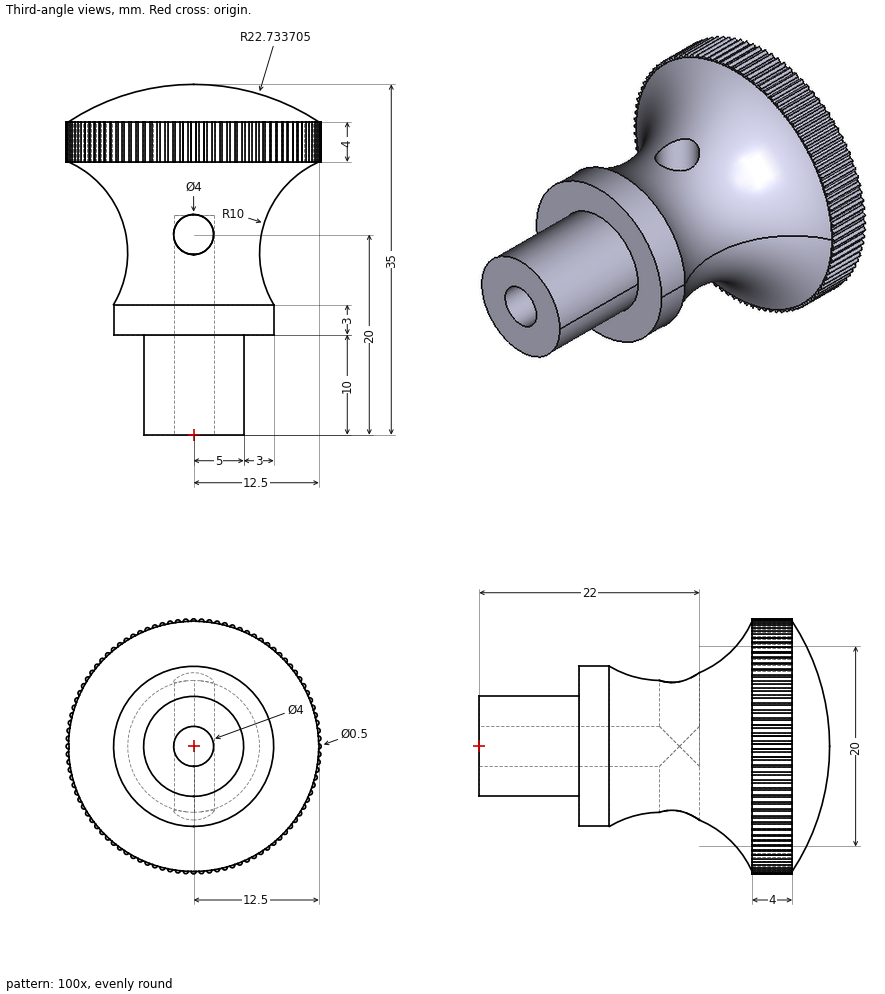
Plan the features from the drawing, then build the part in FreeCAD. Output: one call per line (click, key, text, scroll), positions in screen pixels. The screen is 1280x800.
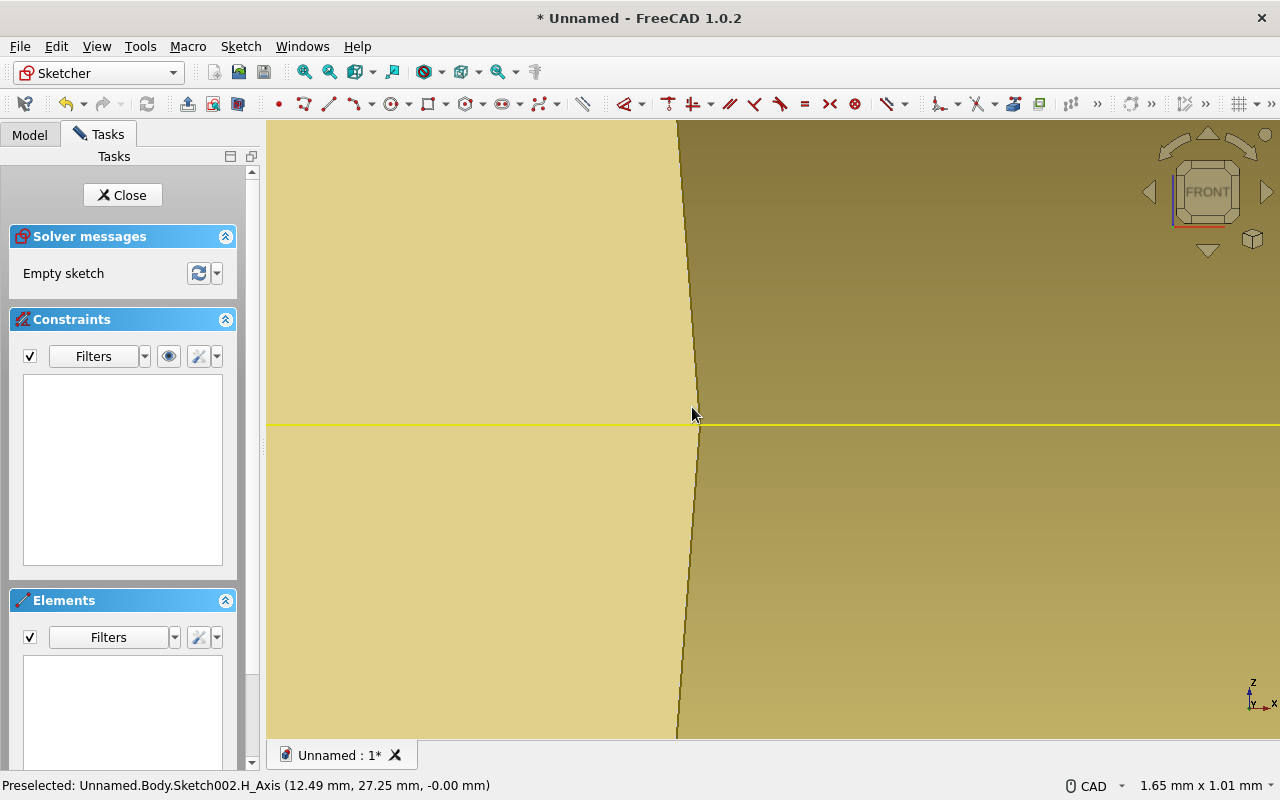
click(390, 104)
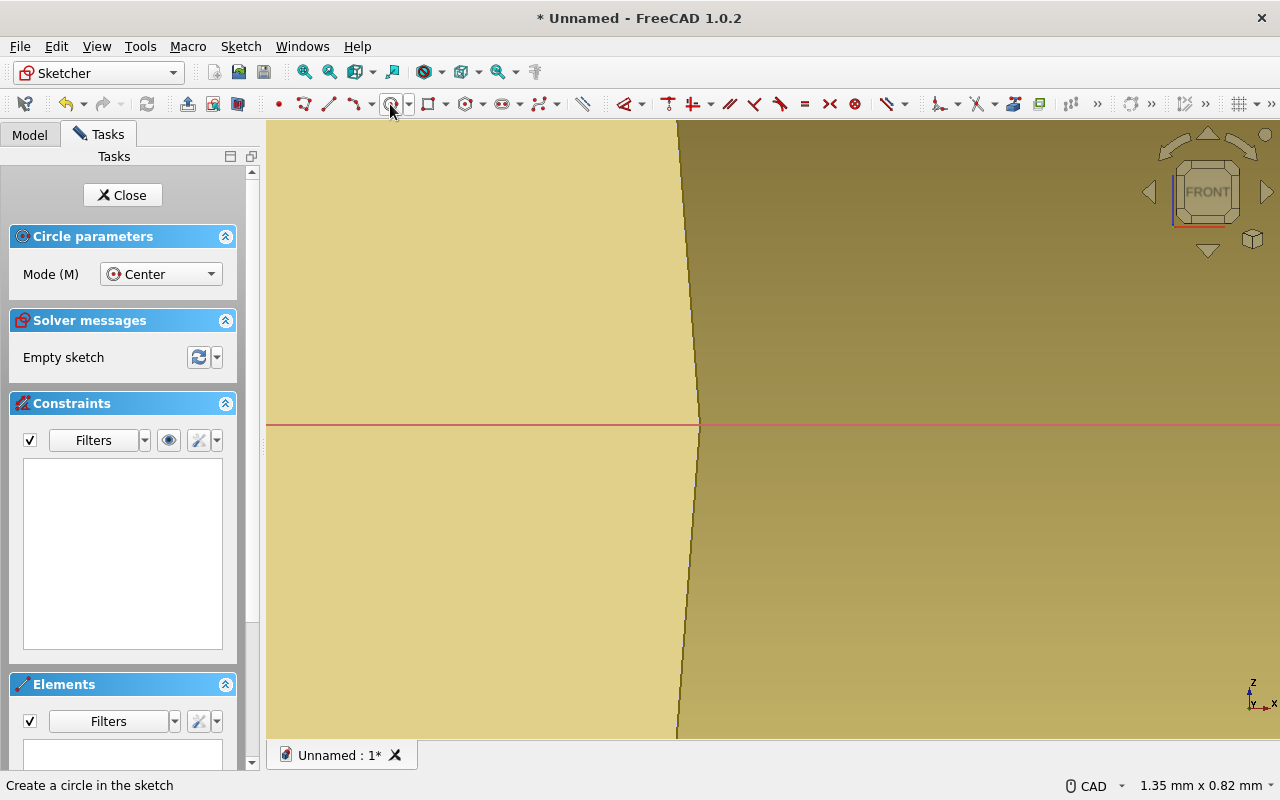
click(700, 425)
move(833, 292)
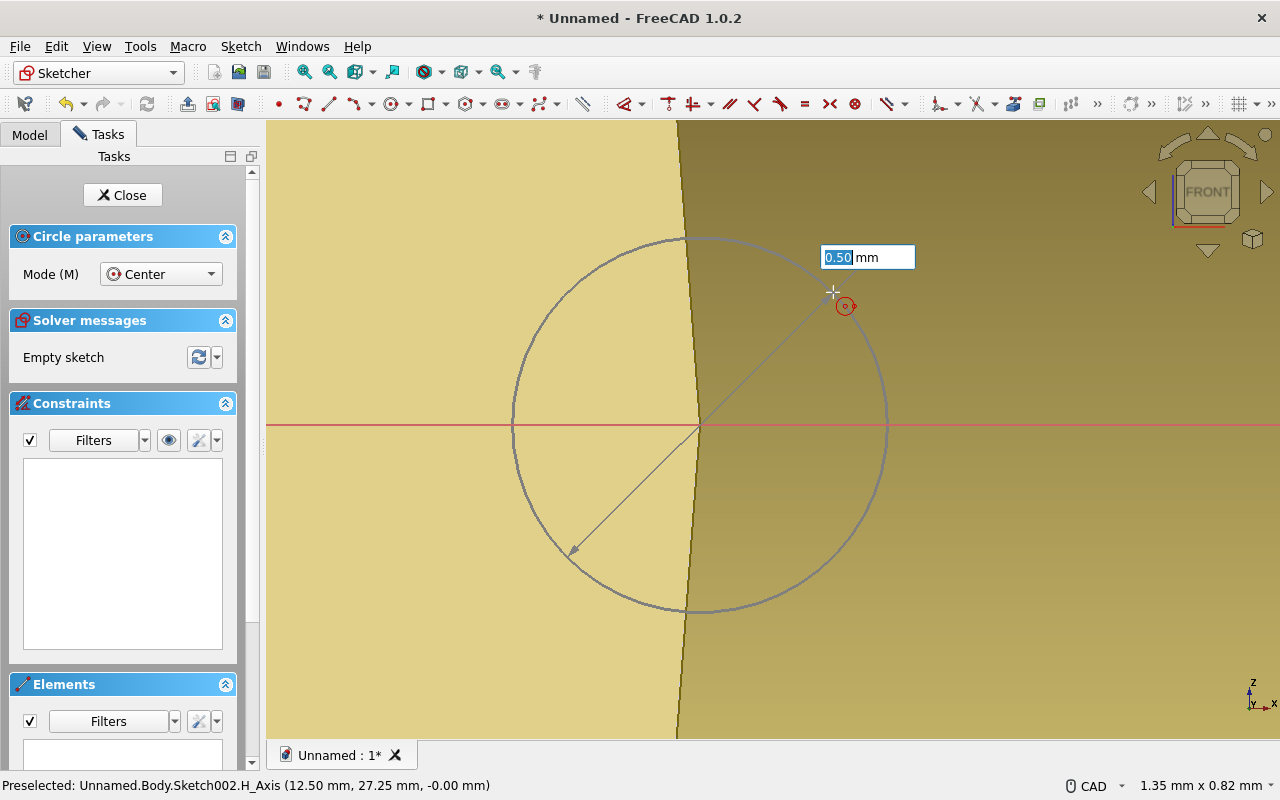
text(0.5)
key(Return)
key(Escape)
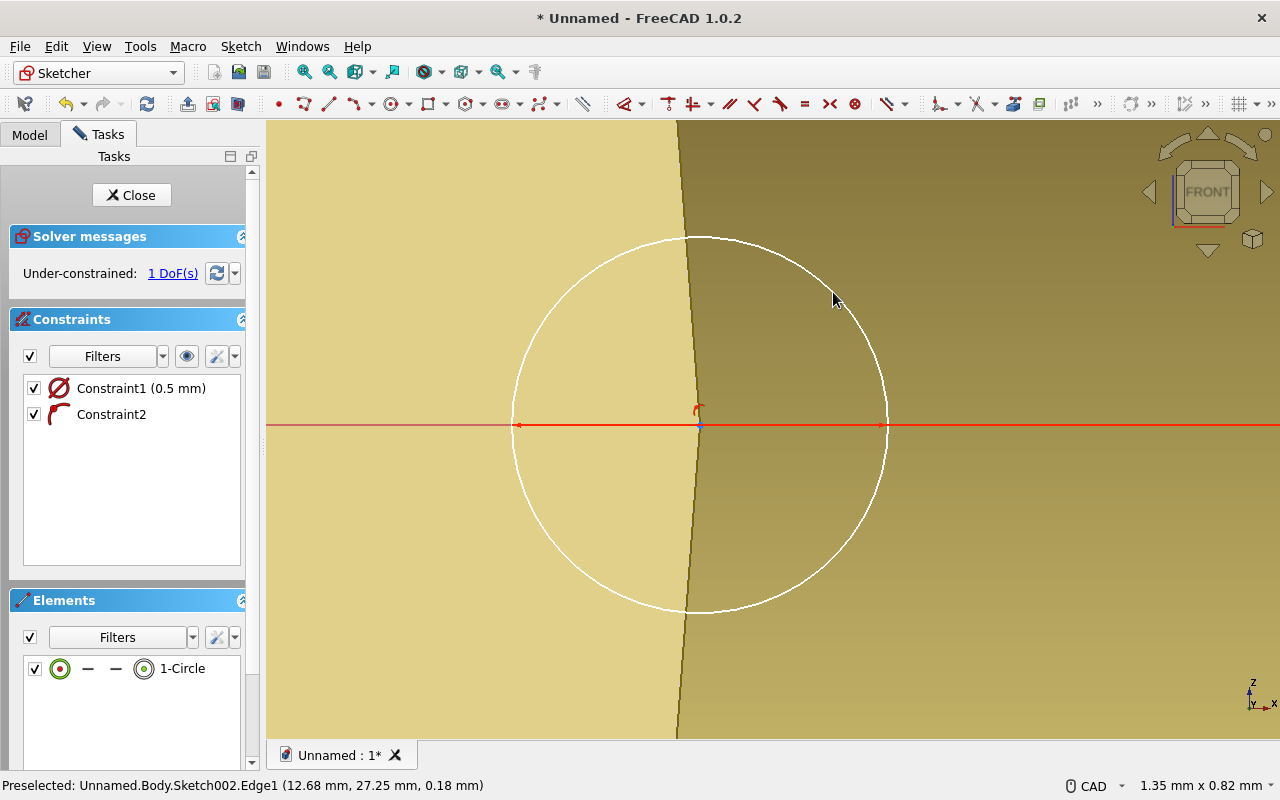
click(624, 104)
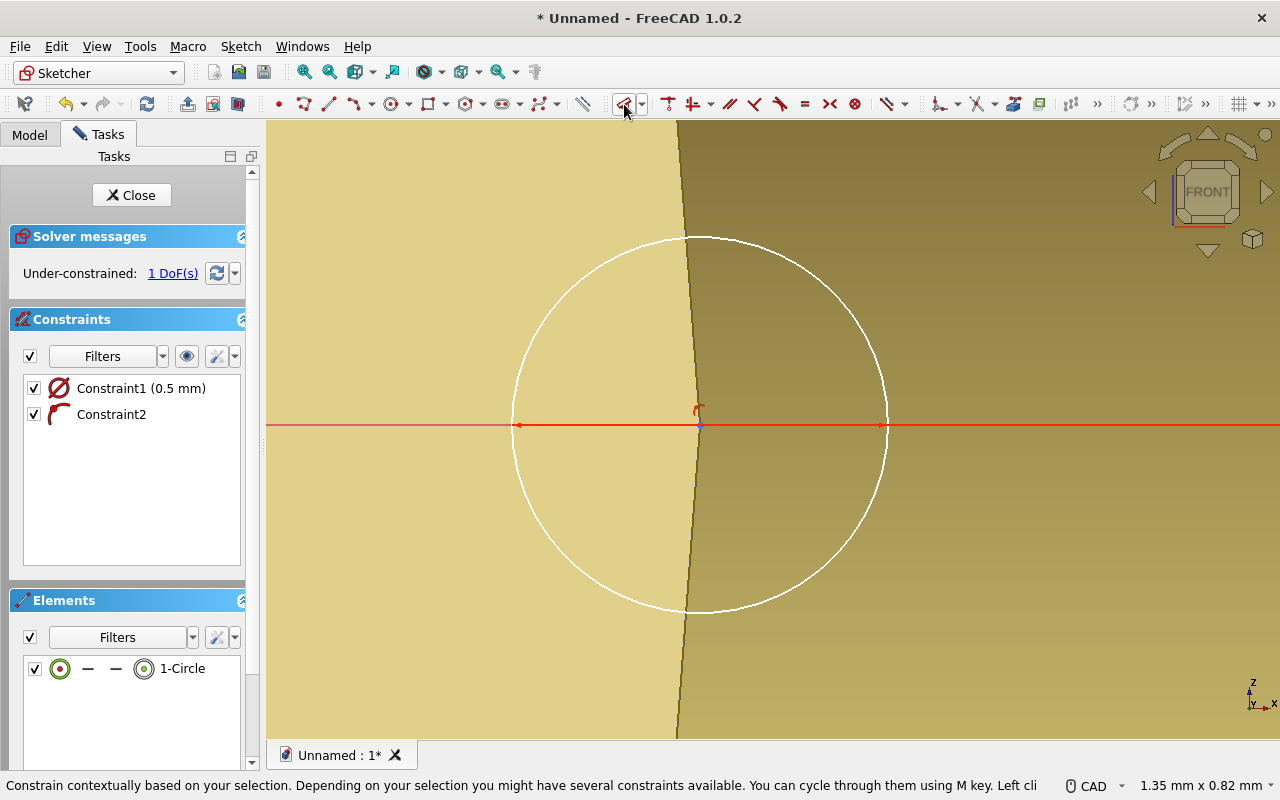
click(700, 425)
click(497, 459)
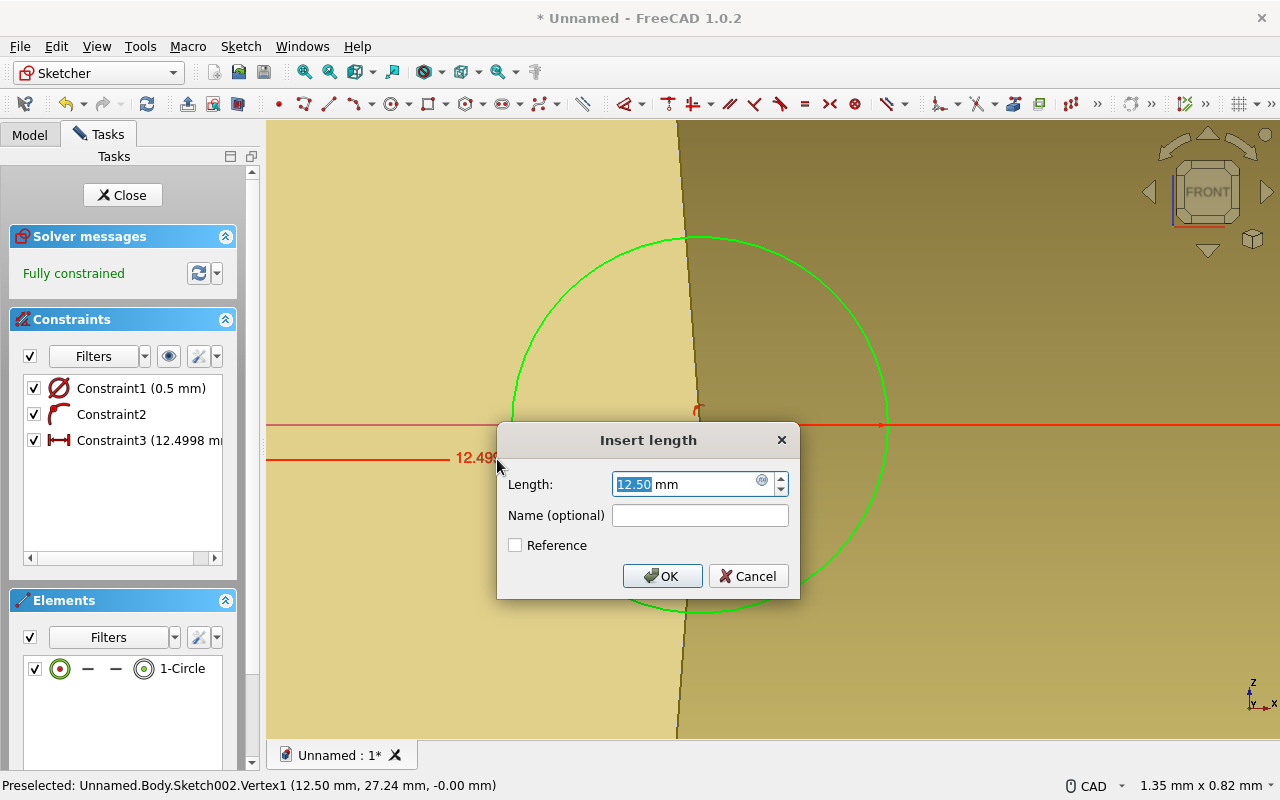
text(12.5)
key(Return)
key(Escape)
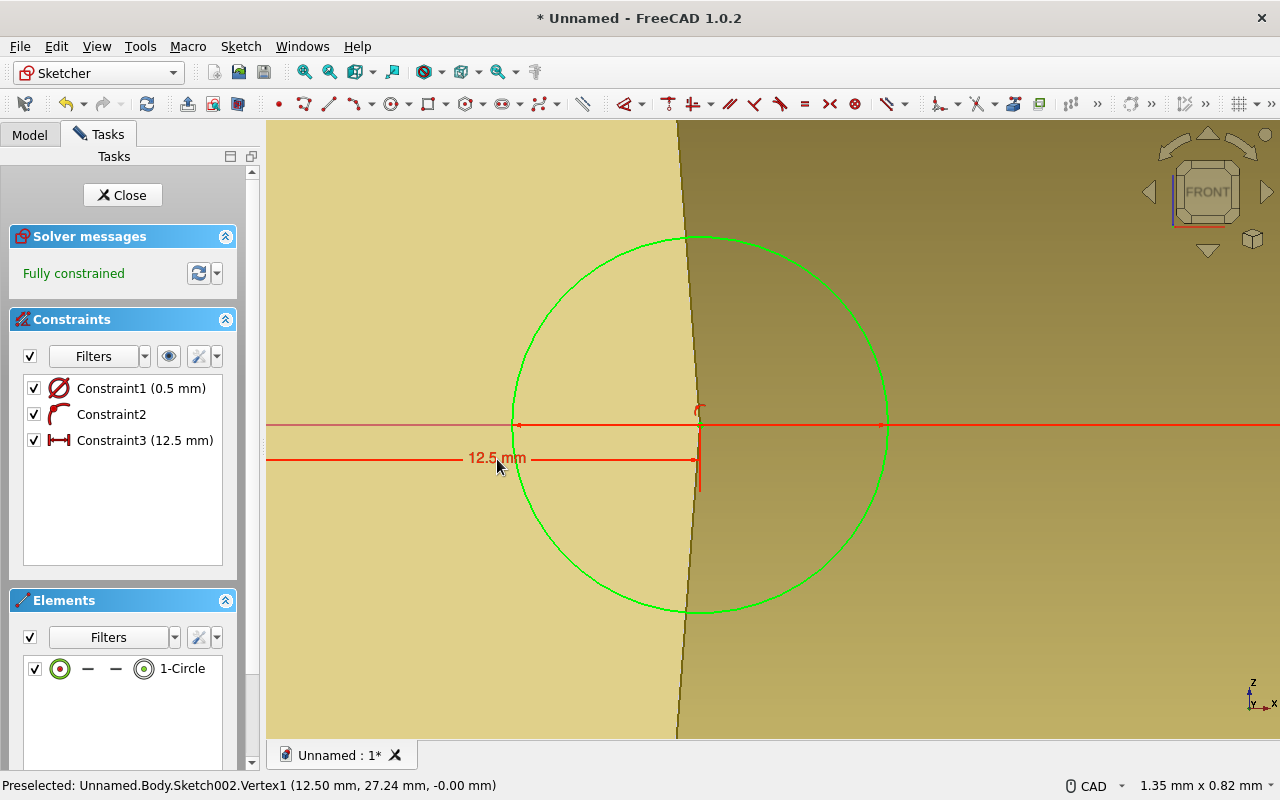
click(123, 195)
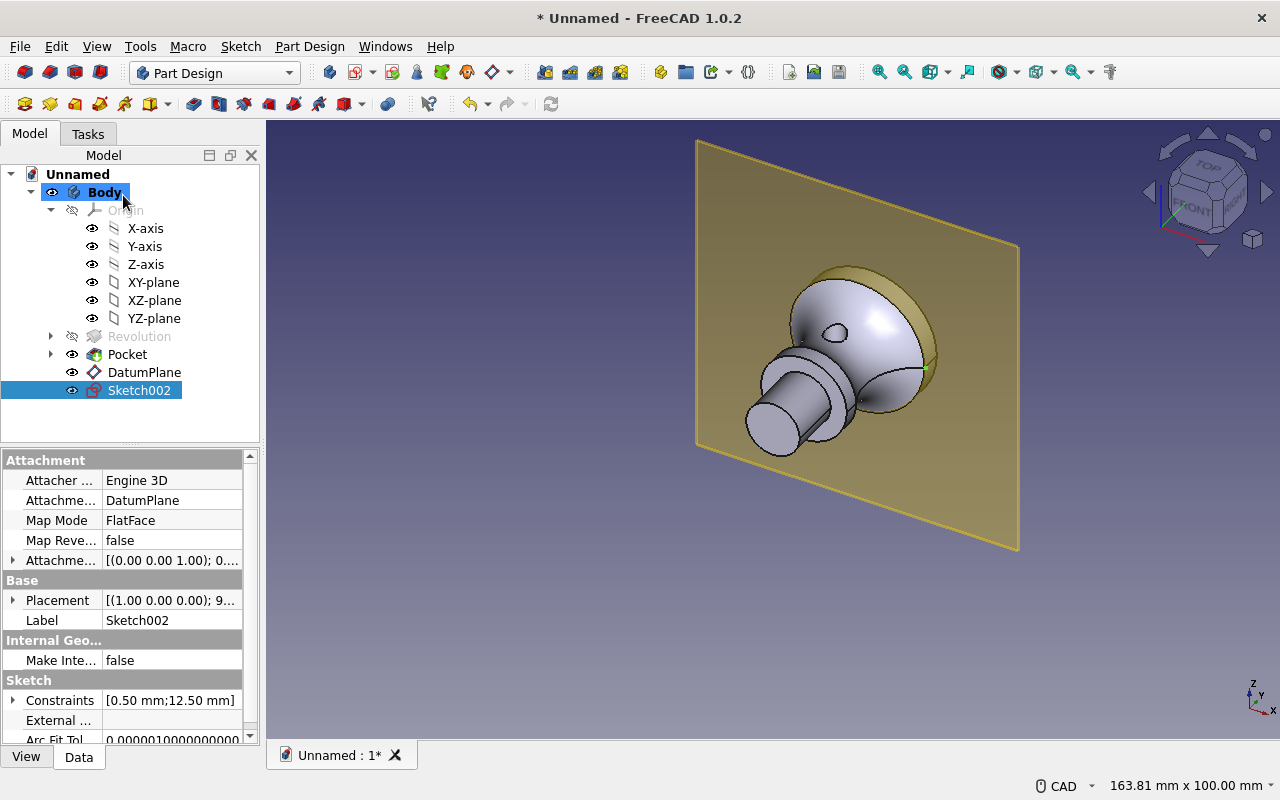
click(25, 104)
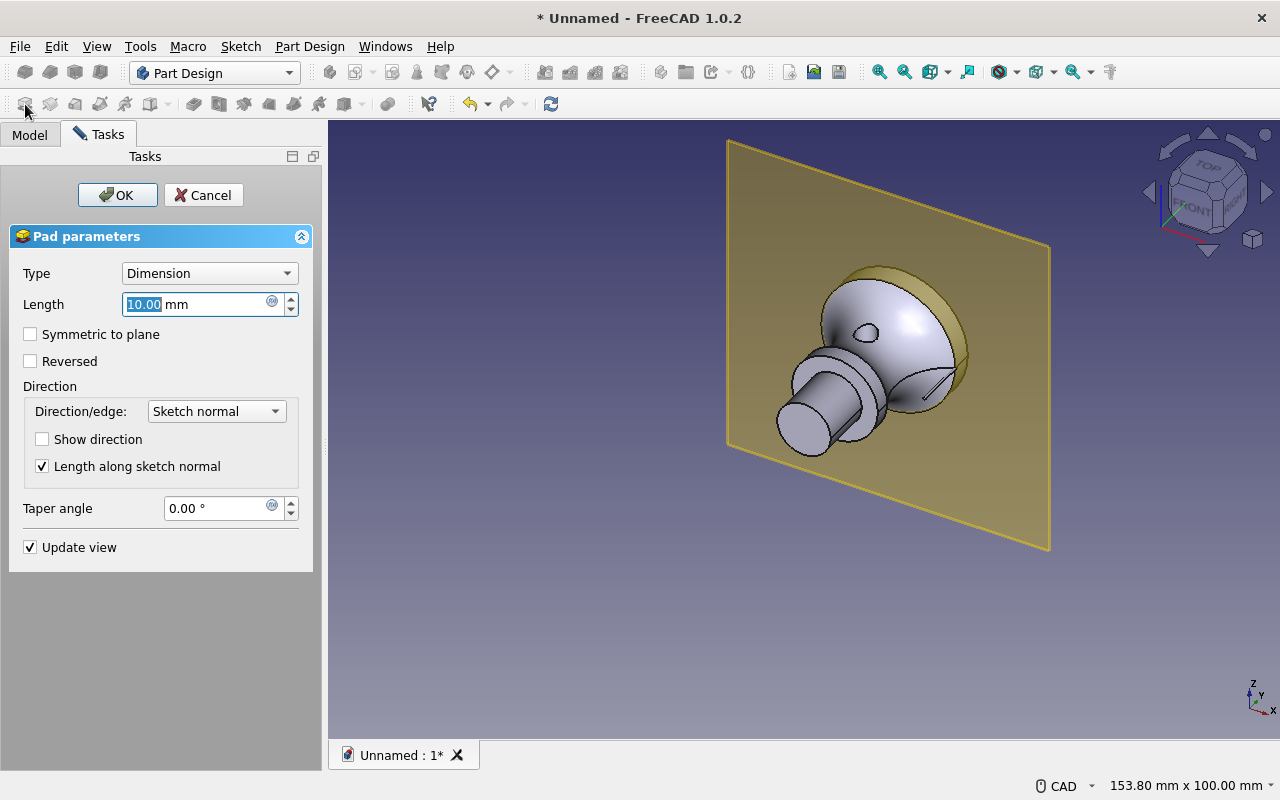
text(4)
key(Tab)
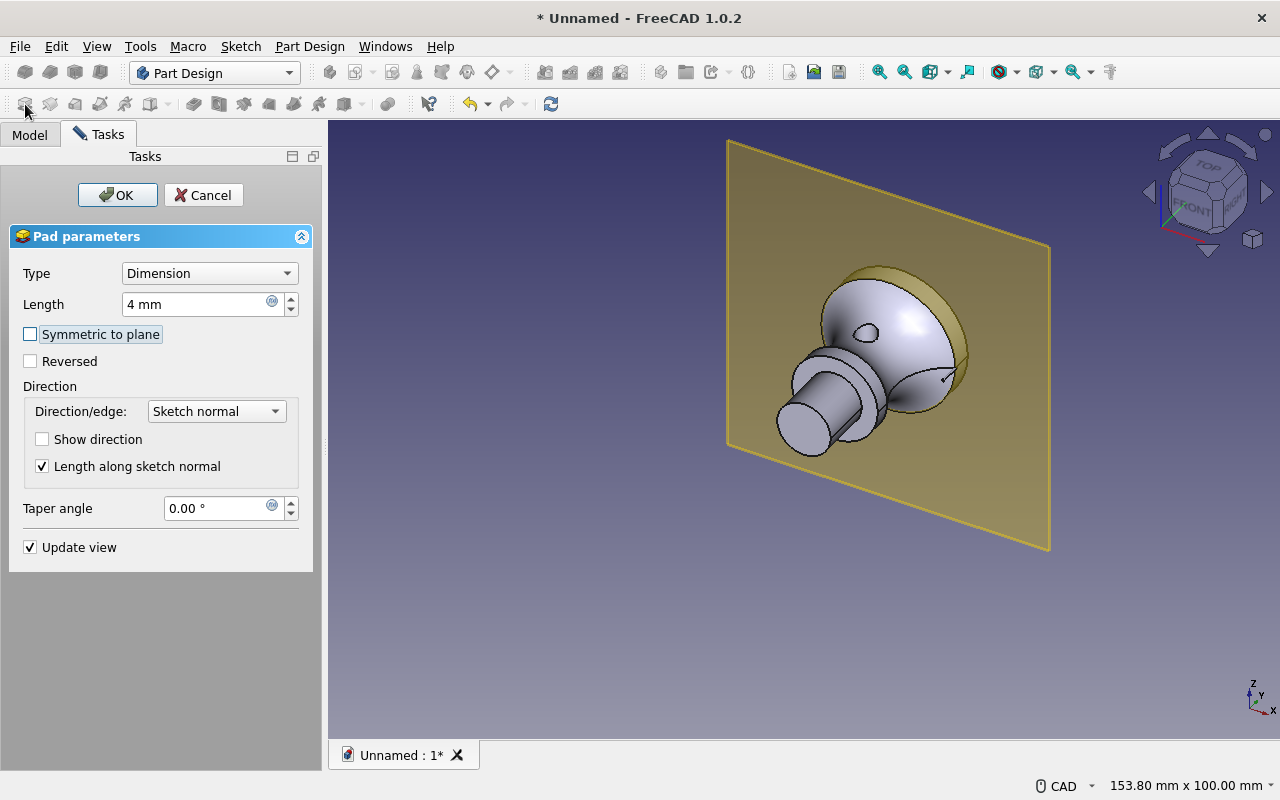
click(31, 361)